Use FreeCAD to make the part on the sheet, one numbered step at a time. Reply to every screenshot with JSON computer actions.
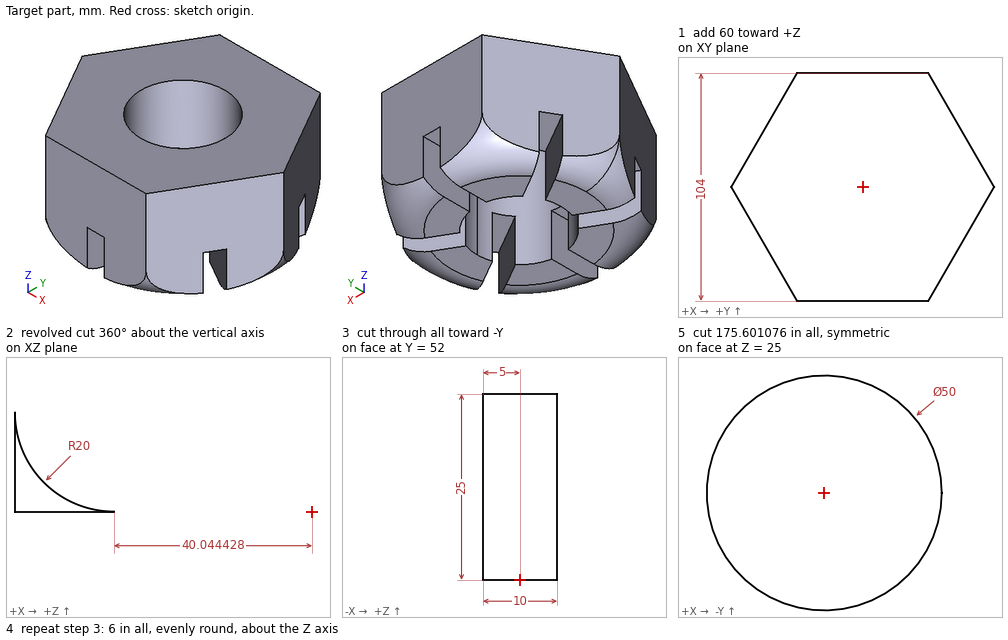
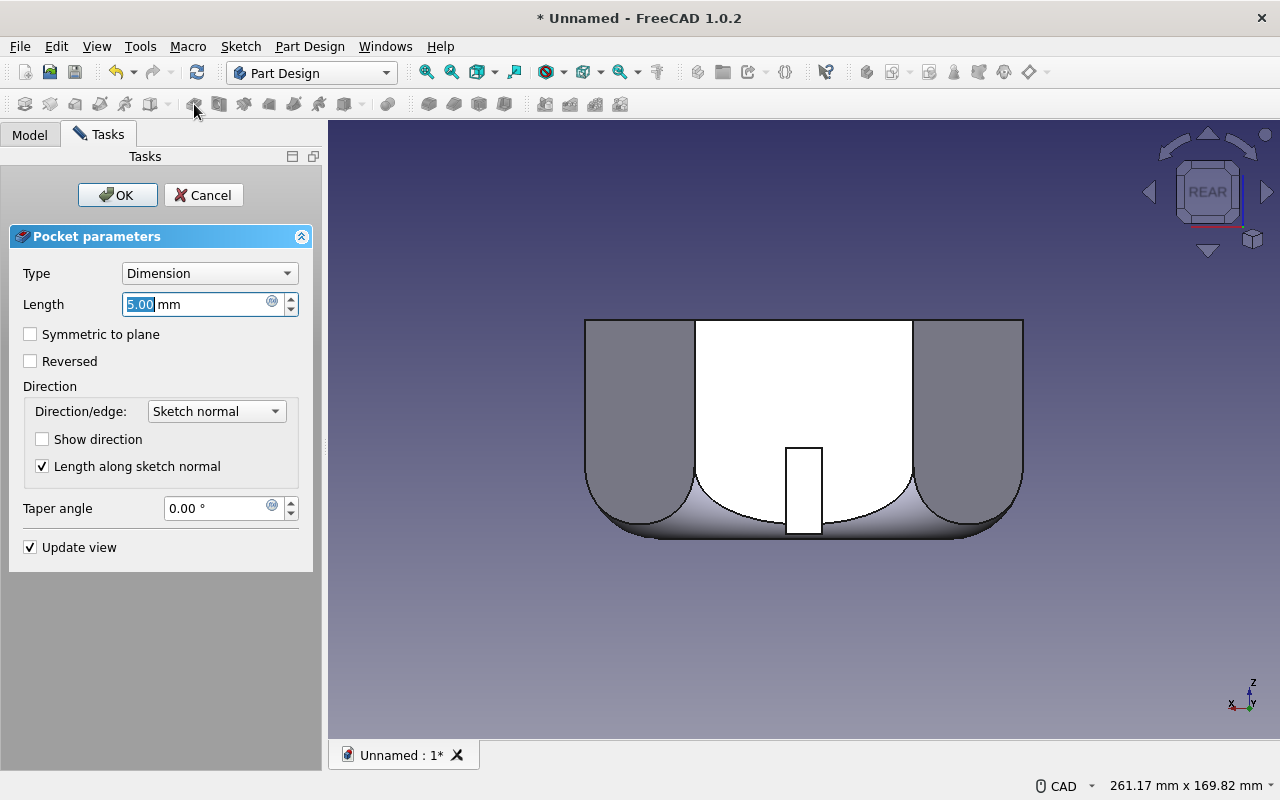
{"action": "left_click", "coordinate": [210, 274]}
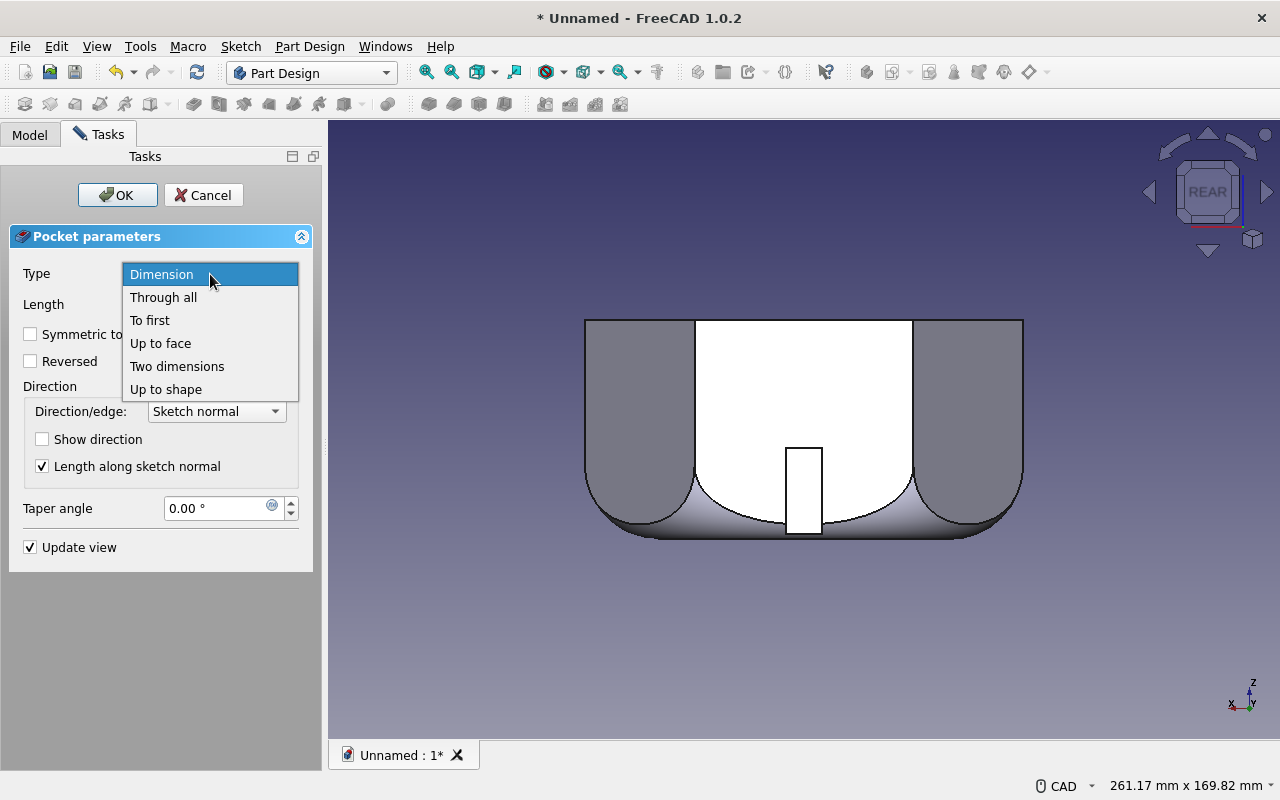
{"action": "left_click", "coordinate": [208, 298]}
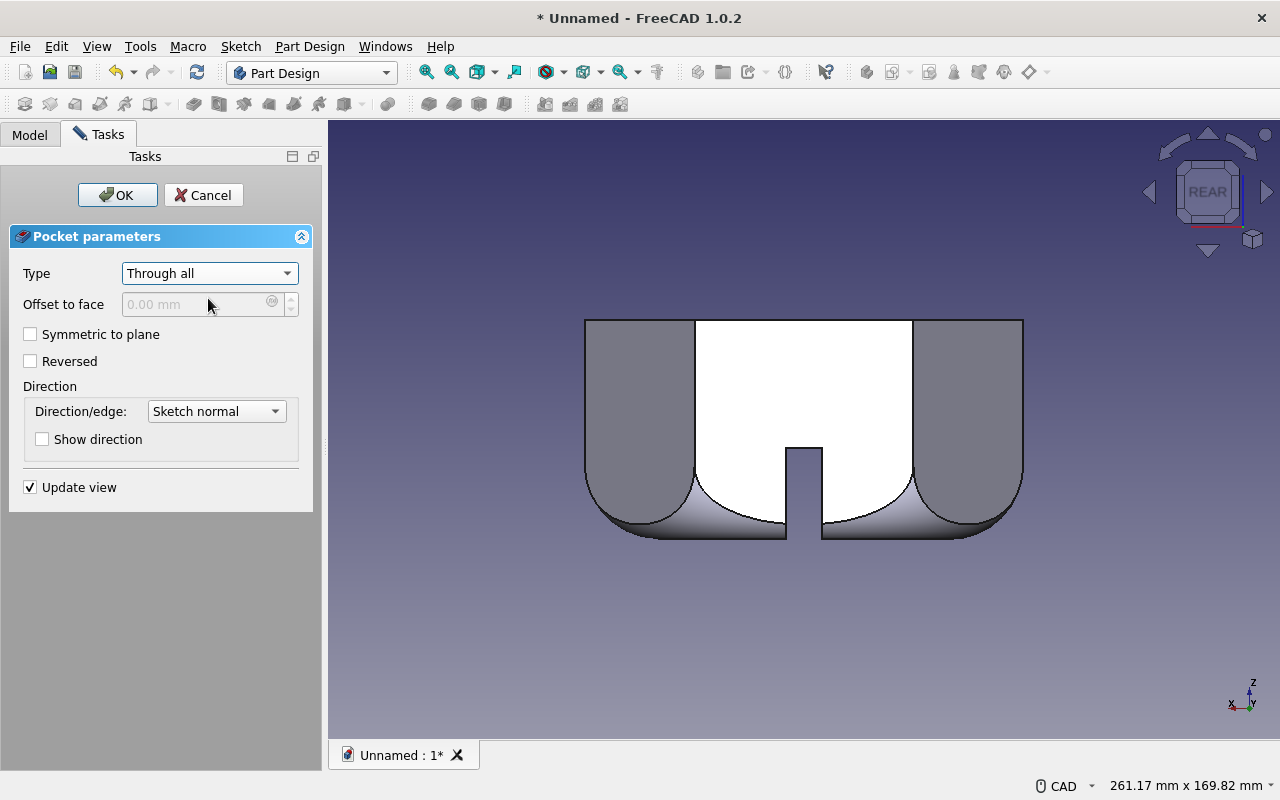
{"action": "left_click", "coordinate": [118, 195]}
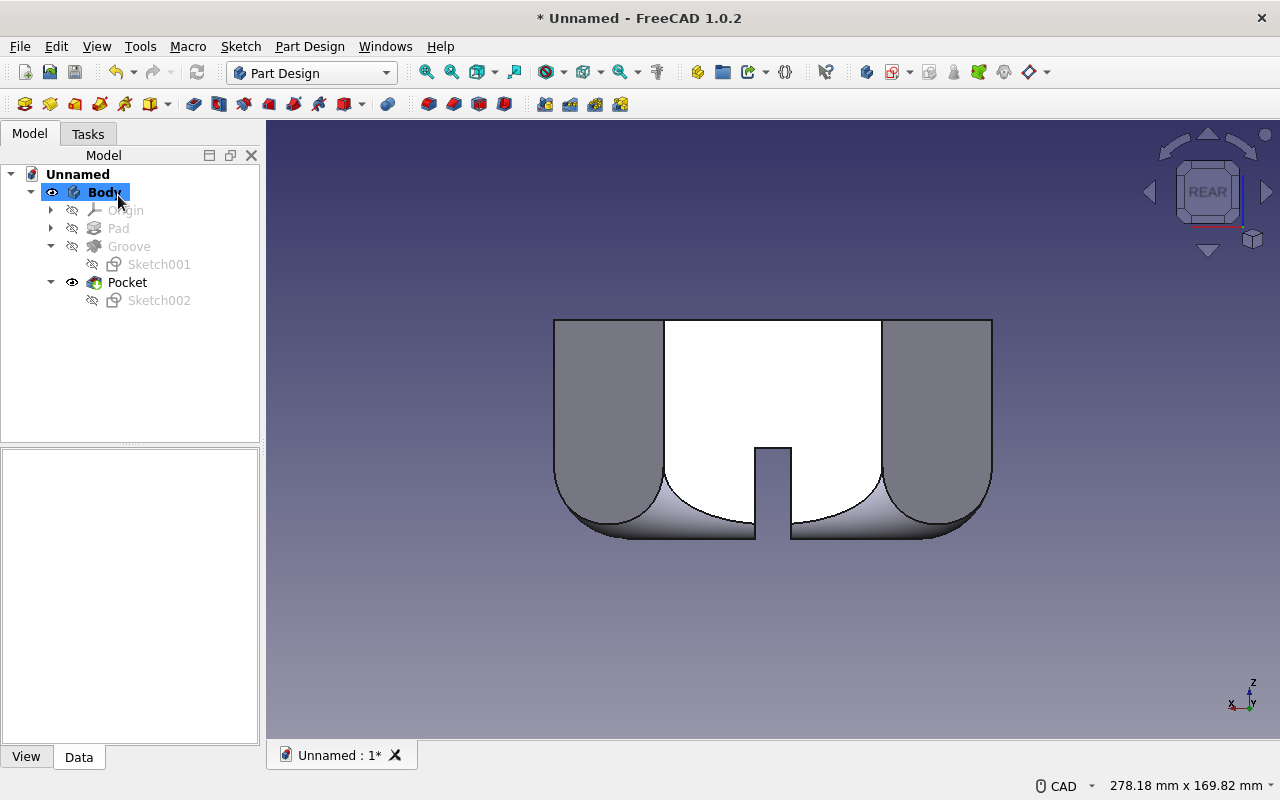
{"action": "left_click", "coordinate": [427, 72]}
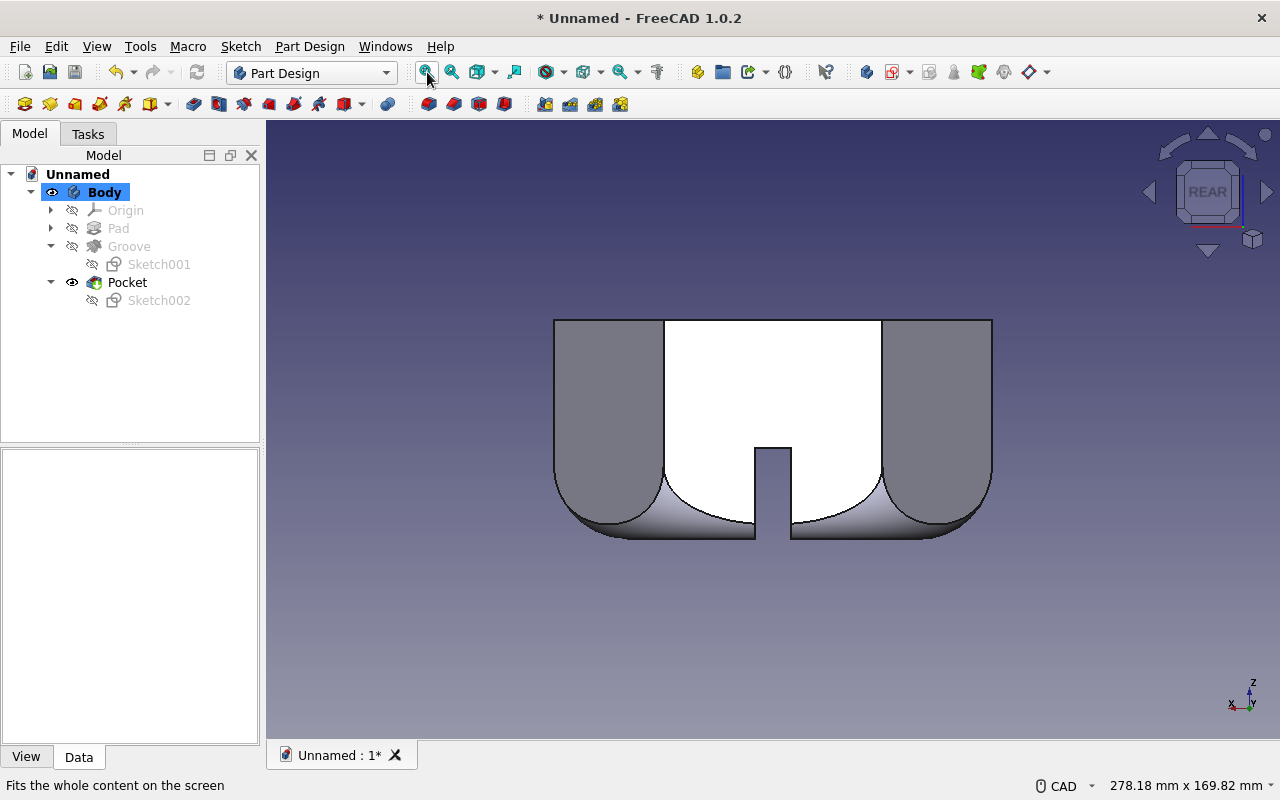
{"action": "left_click", "coordinate": [117, 282]}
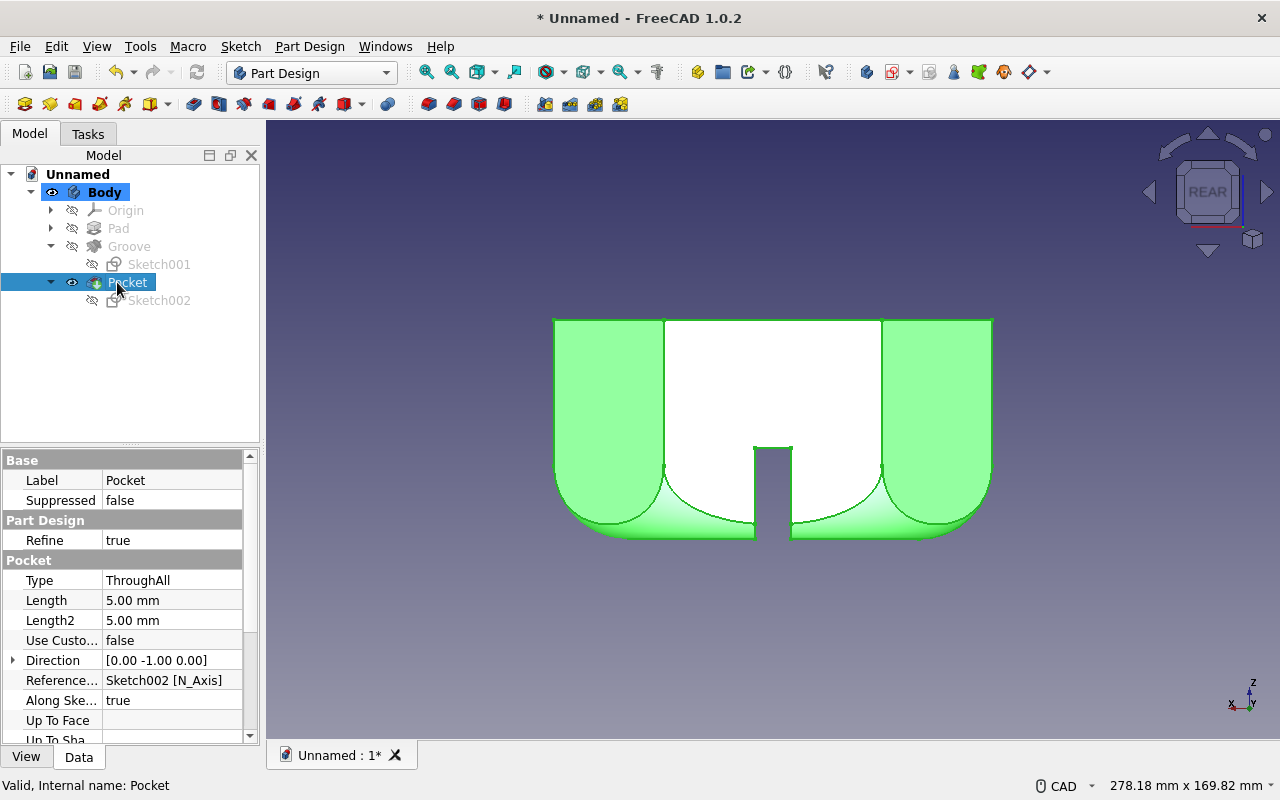
{"action": "left_click", "coordinate": [595, 104]}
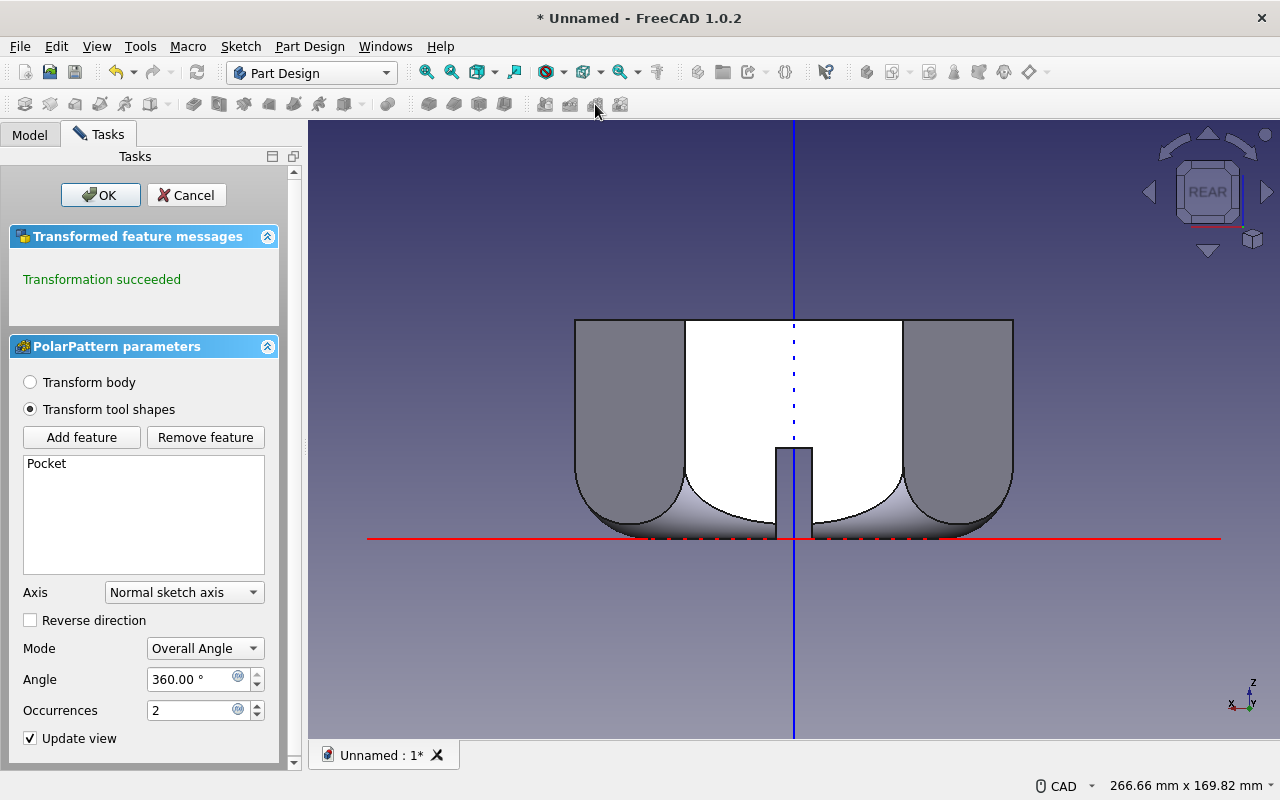
{"action": "left_click", "coordinate": [185, 592]}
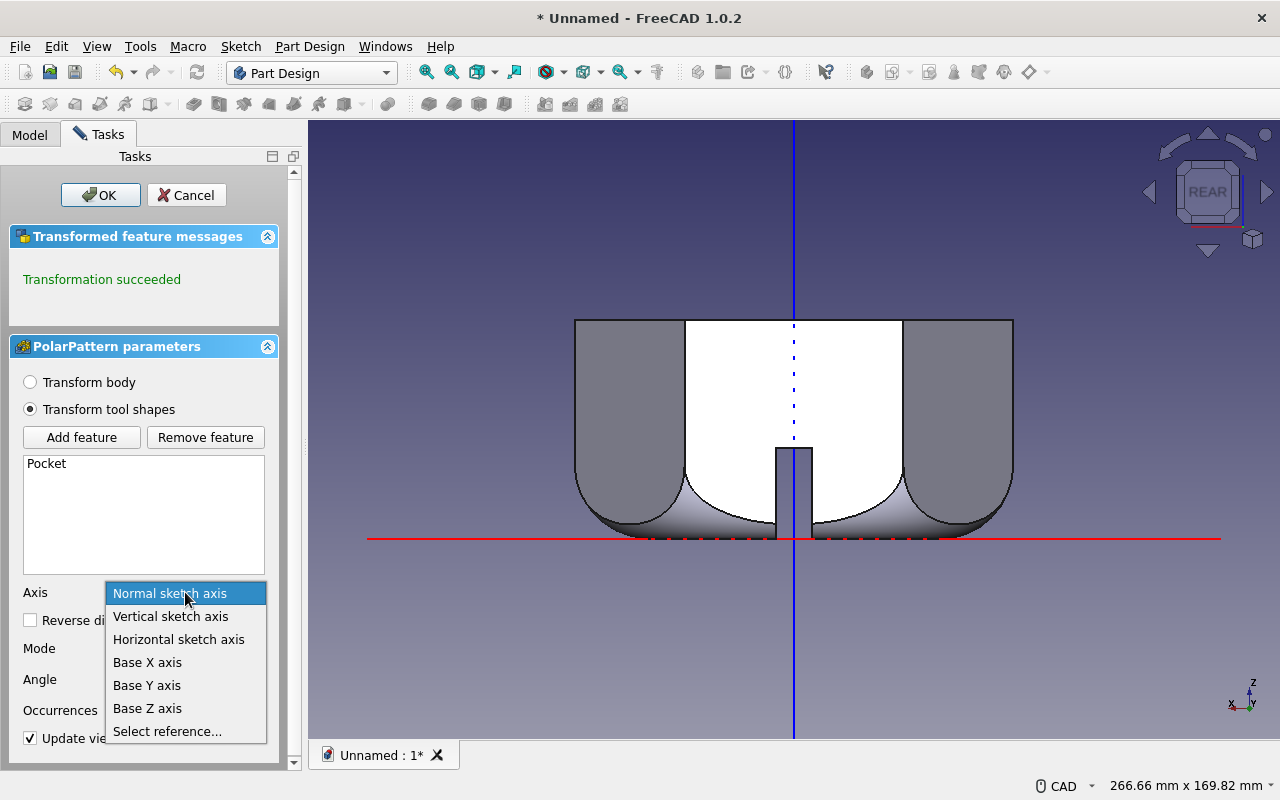
{"action": "left_click", "coordinate": [184, 708]}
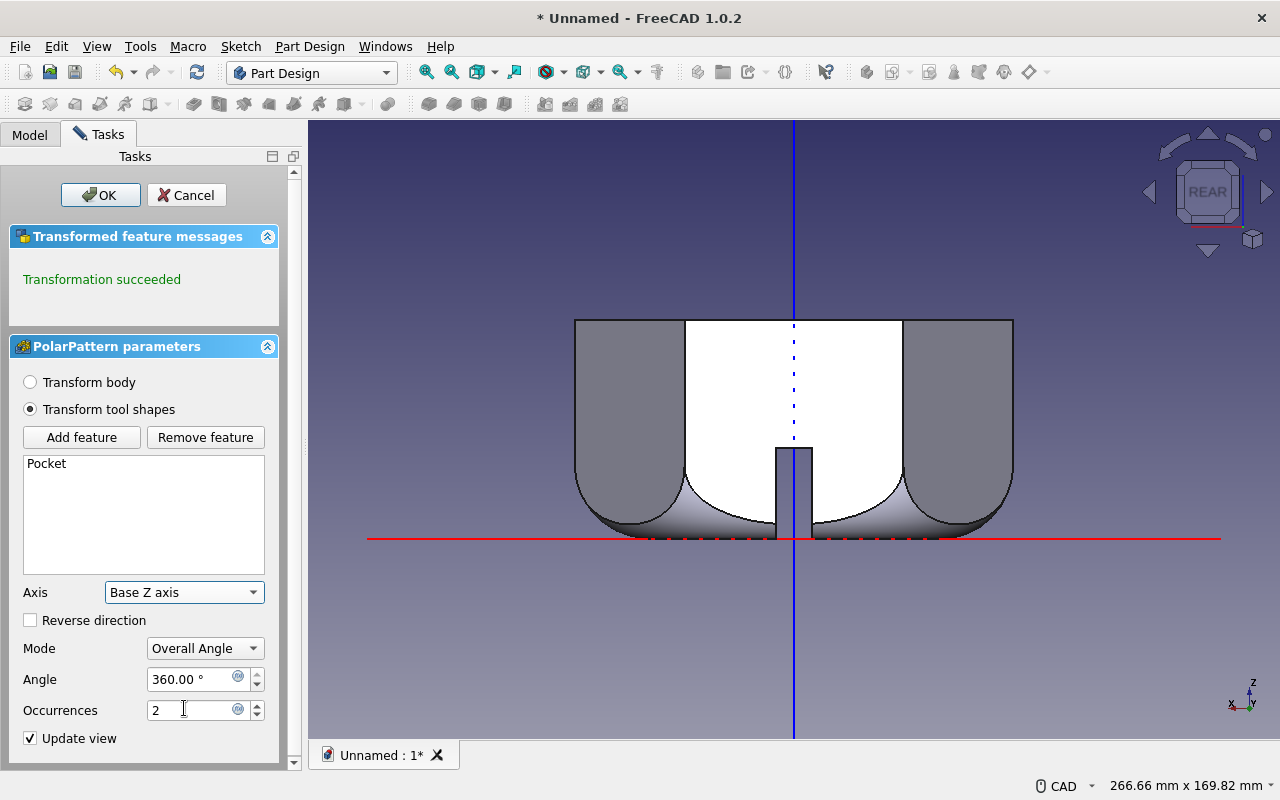
{"action": "triple_click", "coordinate": [199, 710]}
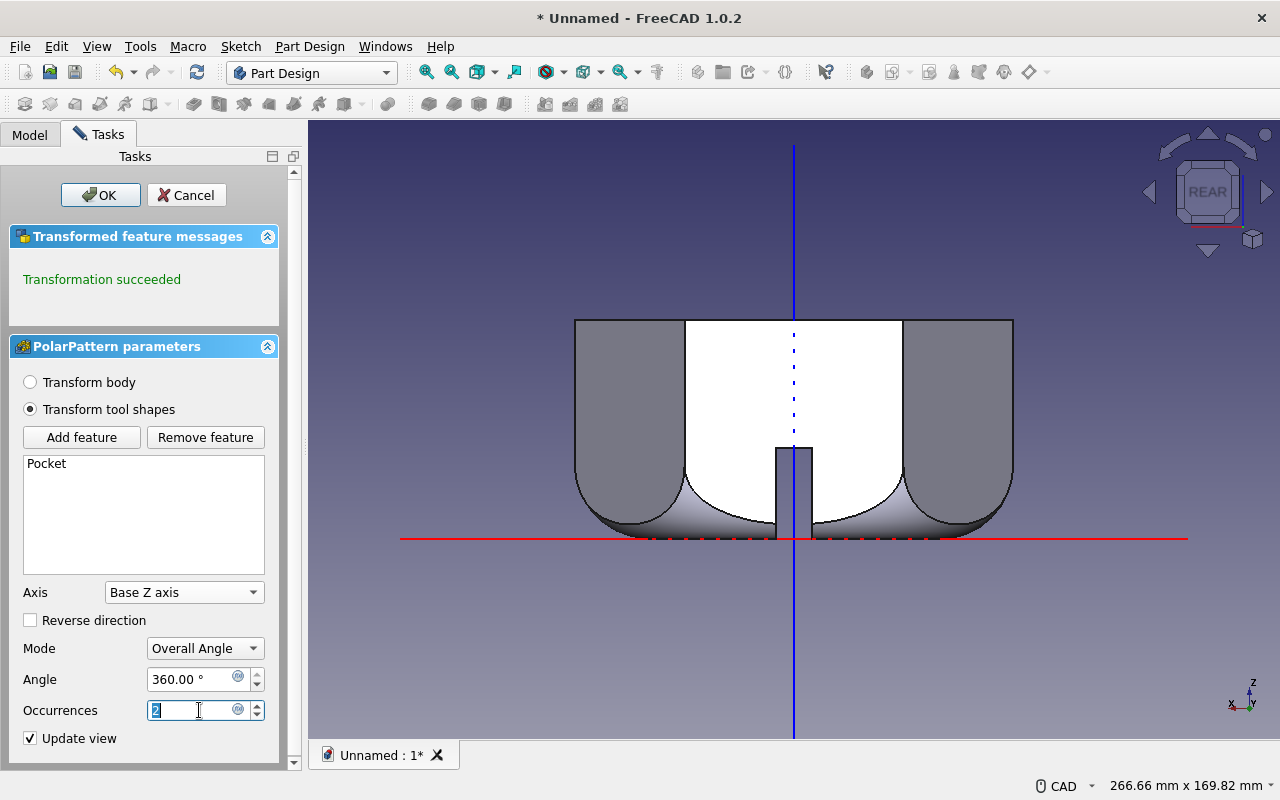
{"action": "type", "text": "6"}
{"action": "key", "text": "Tab"}